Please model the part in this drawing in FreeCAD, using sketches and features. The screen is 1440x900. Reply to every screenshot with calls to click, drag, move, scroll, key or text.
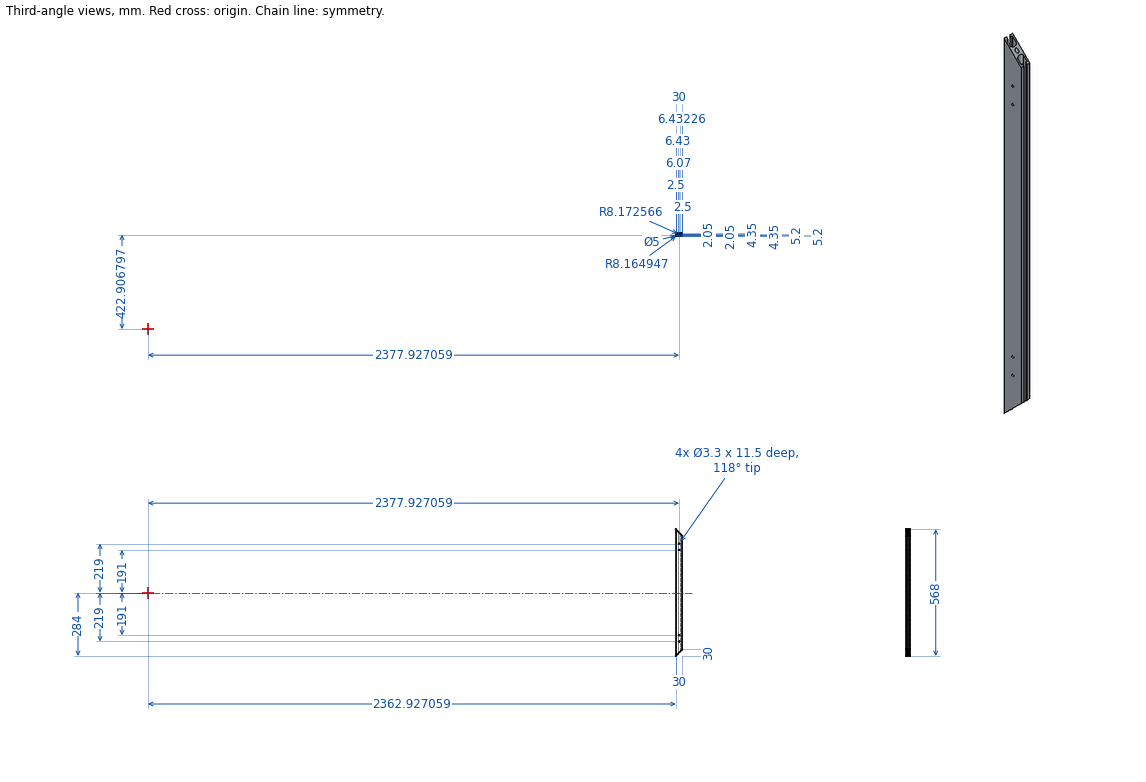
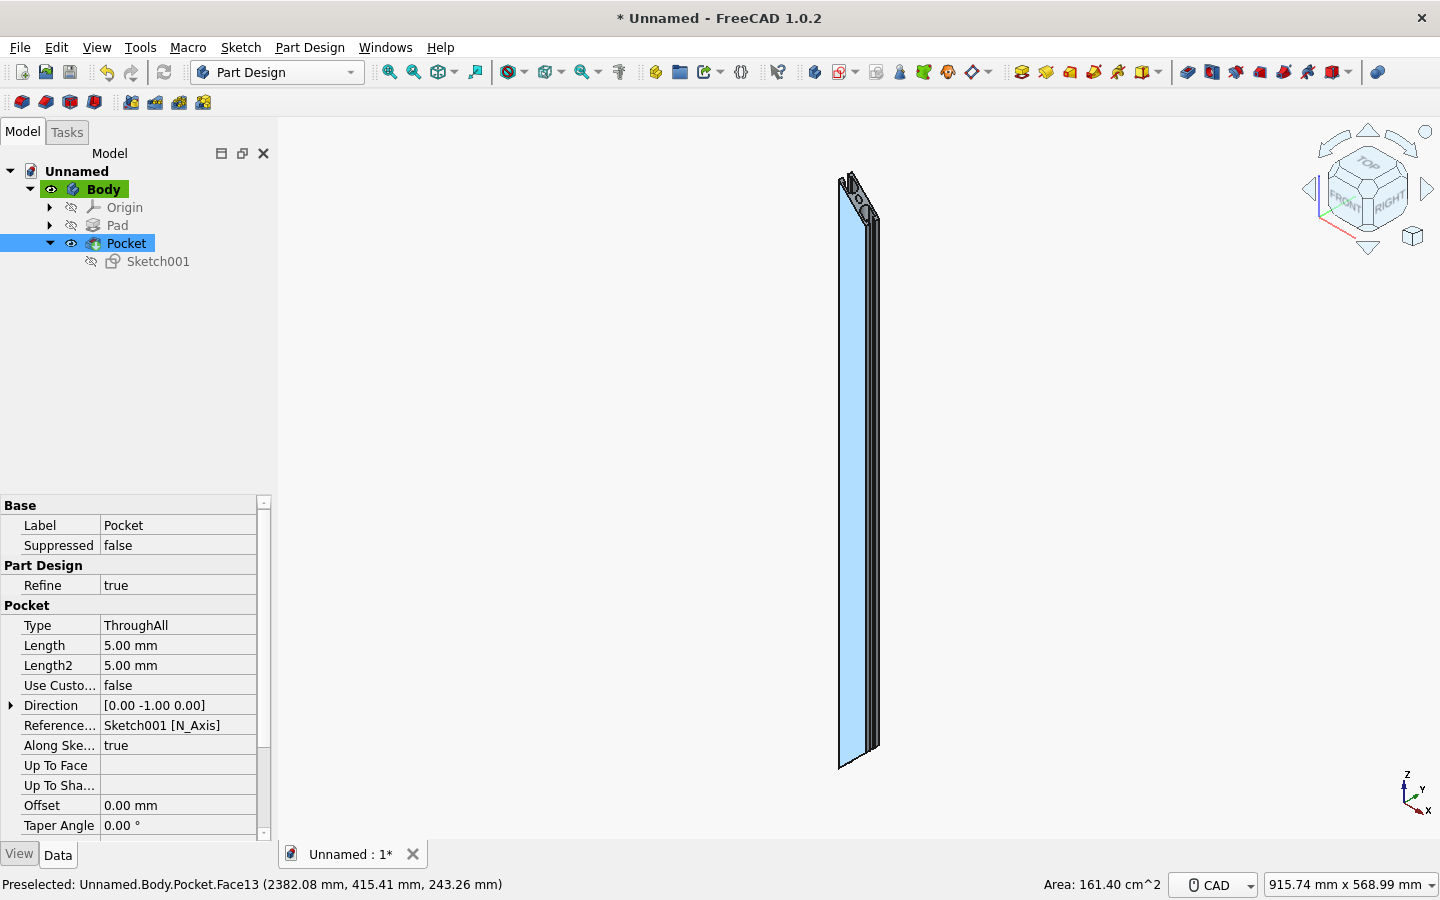
click(840, 72)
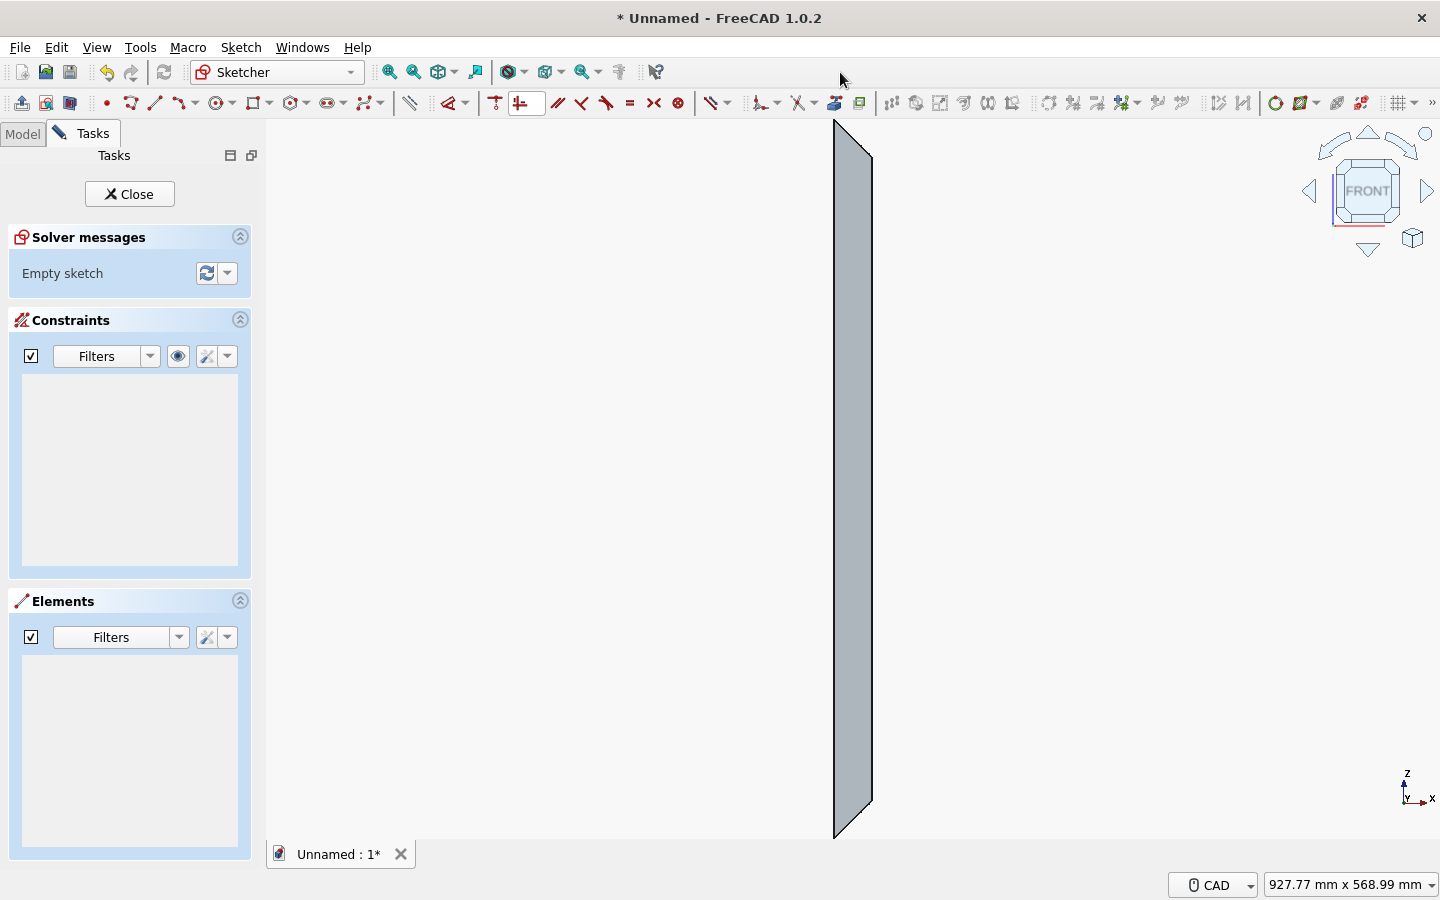
click(216, 104)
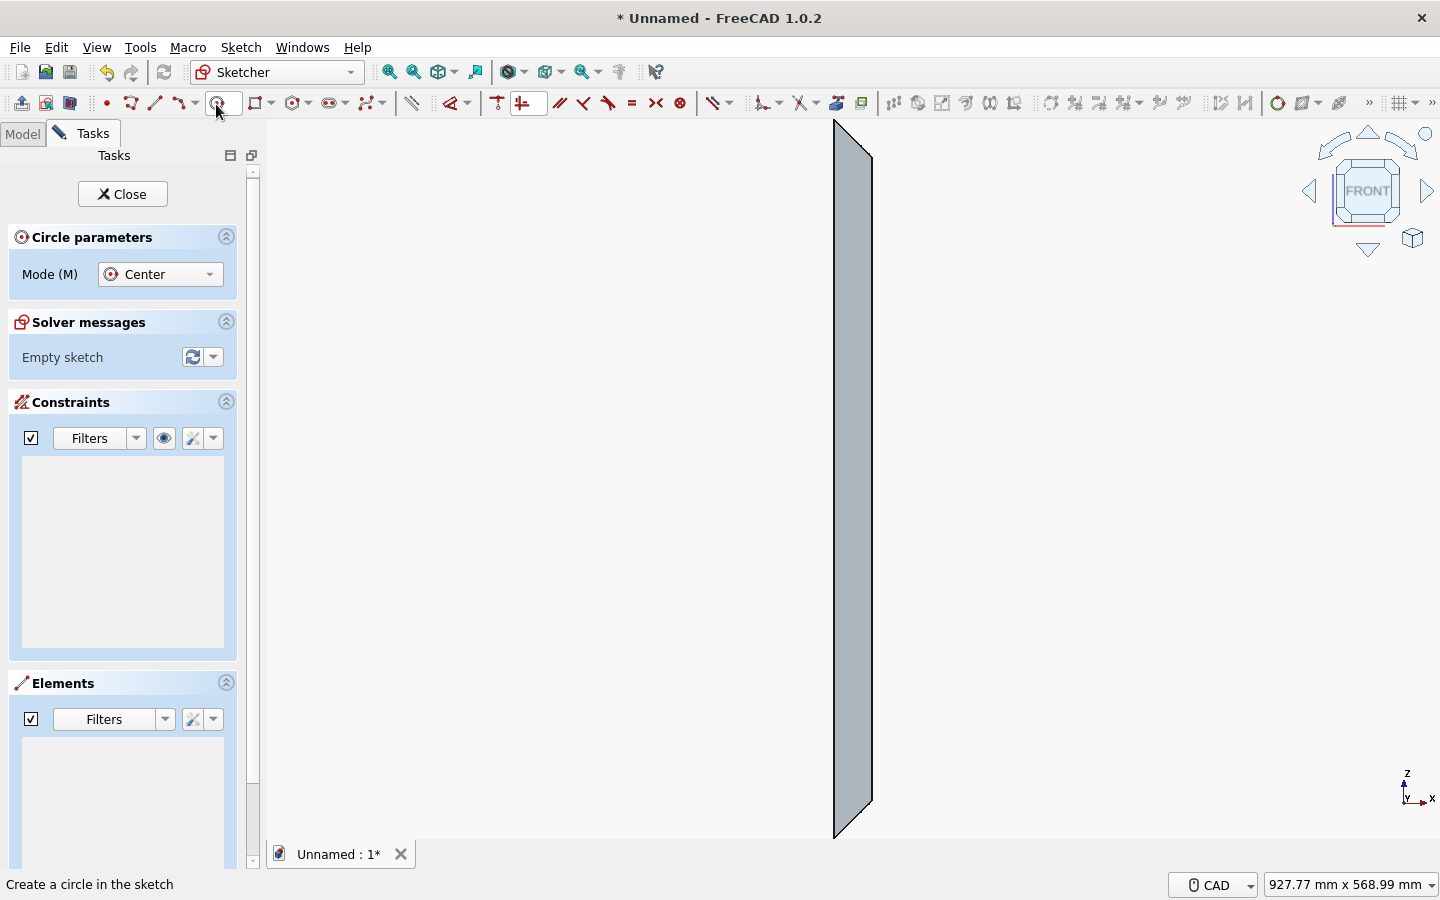
scroll(853, 202, up, 12)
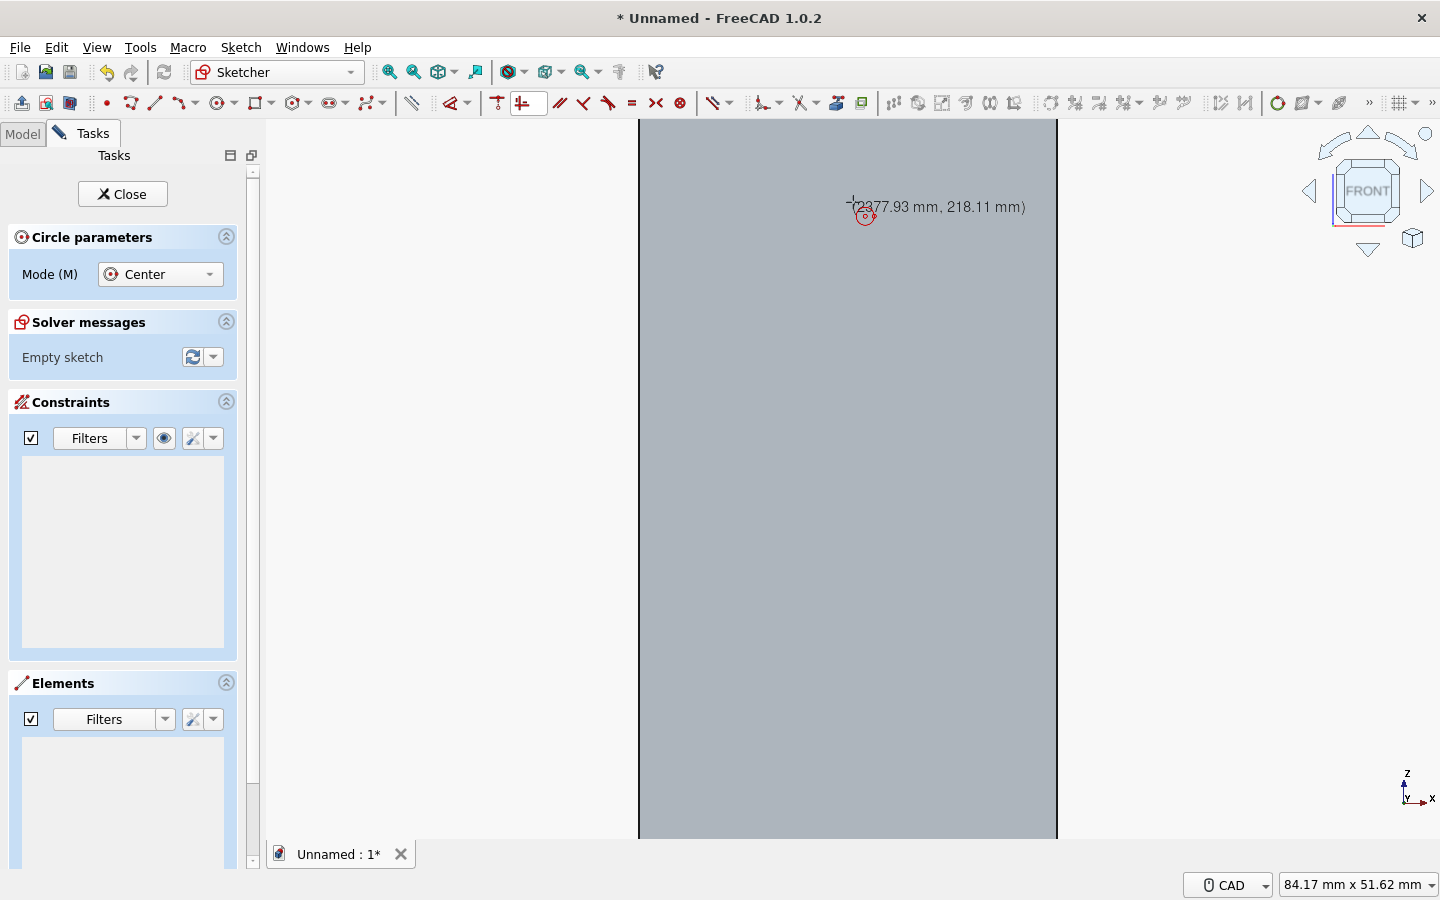
scroll(779, 256, down, 13)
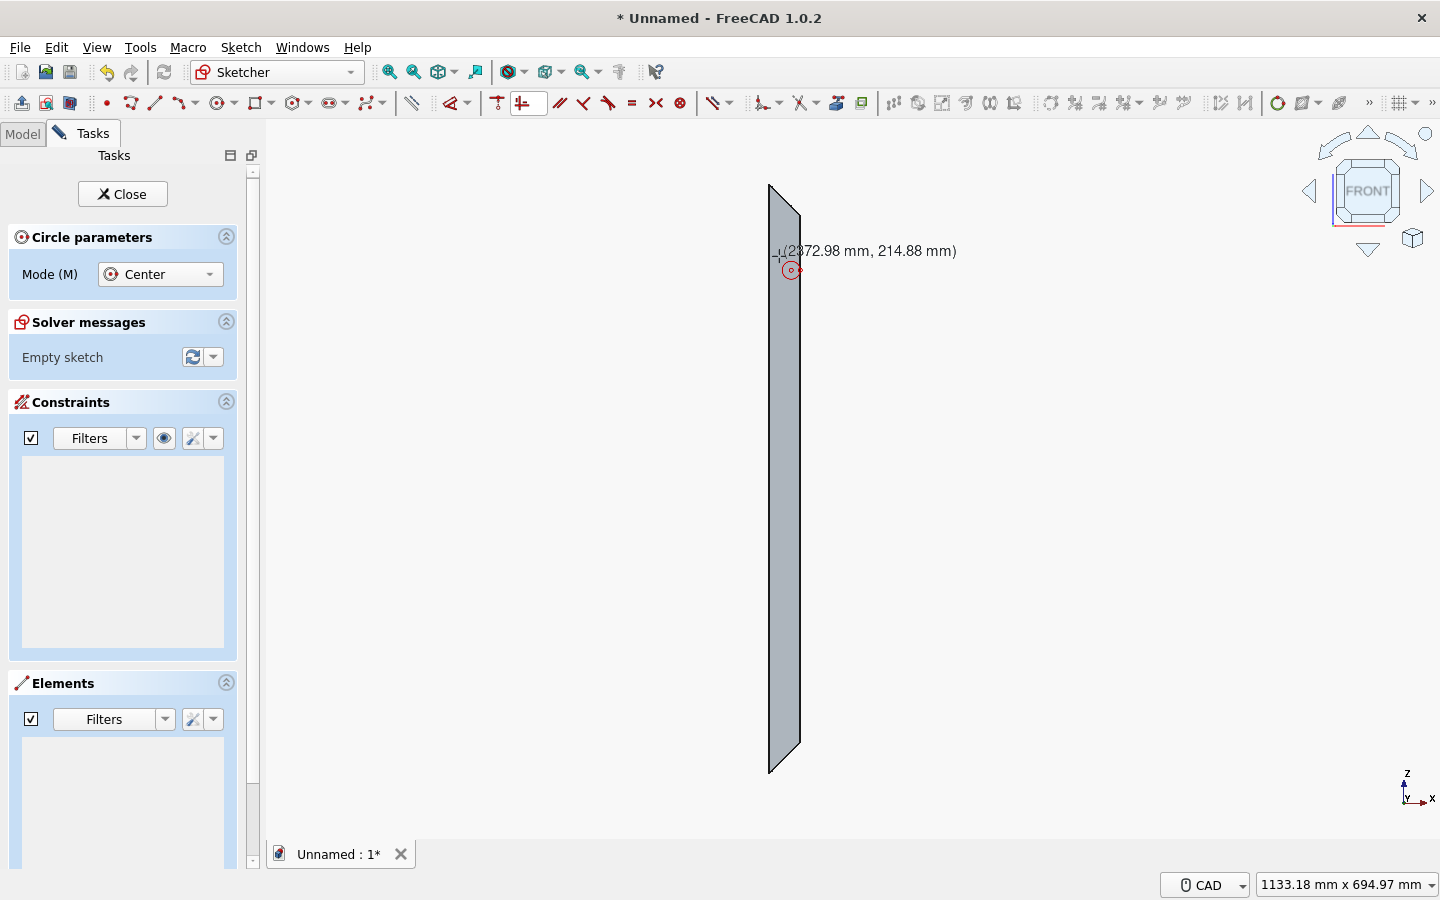
click(785, 252)
move(786, 251)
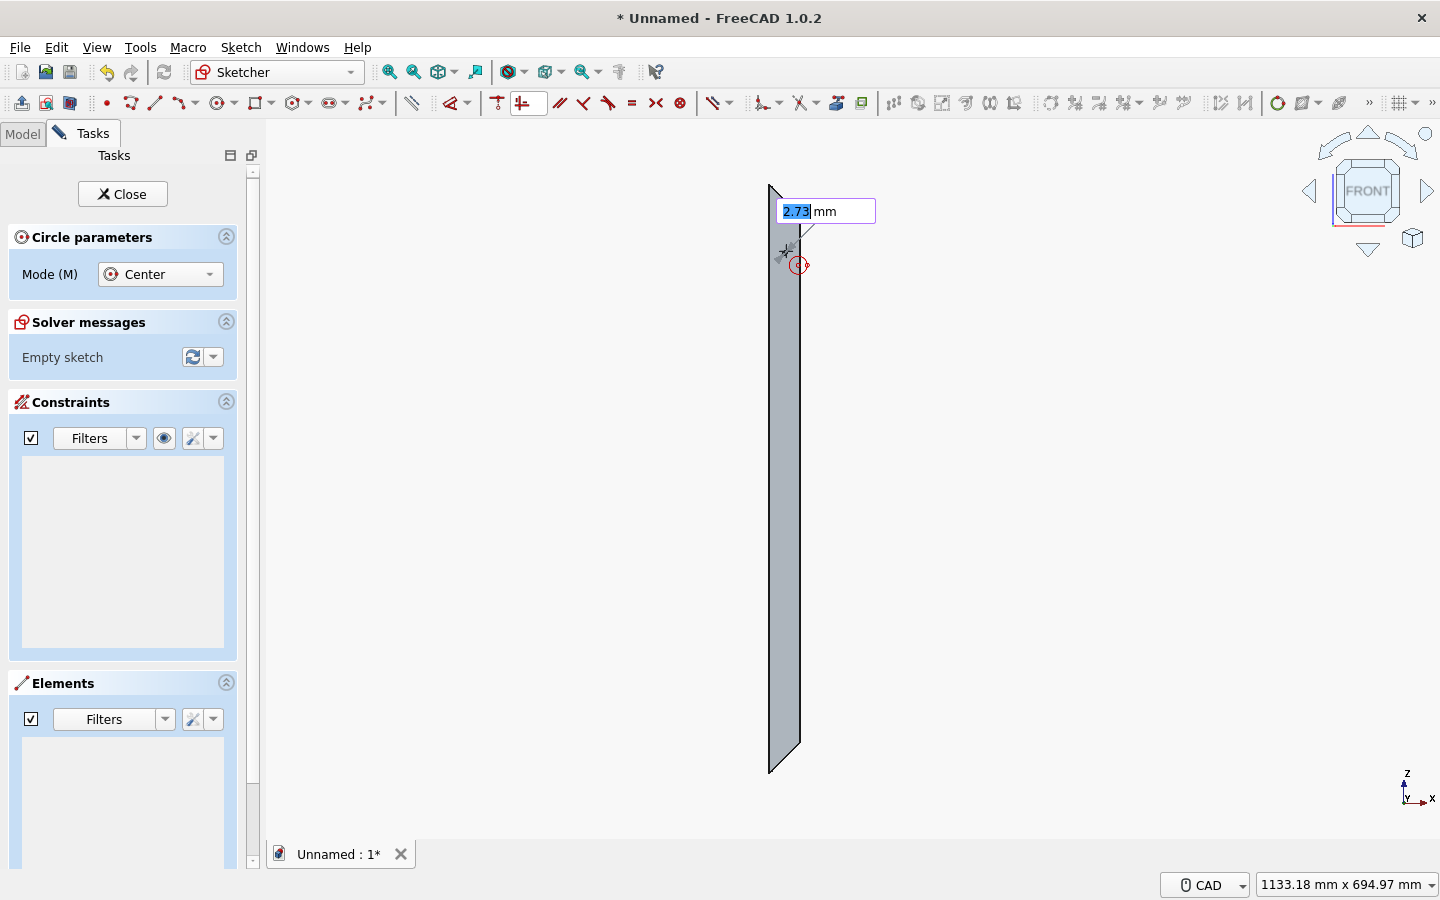
text(3.3)
key(Return)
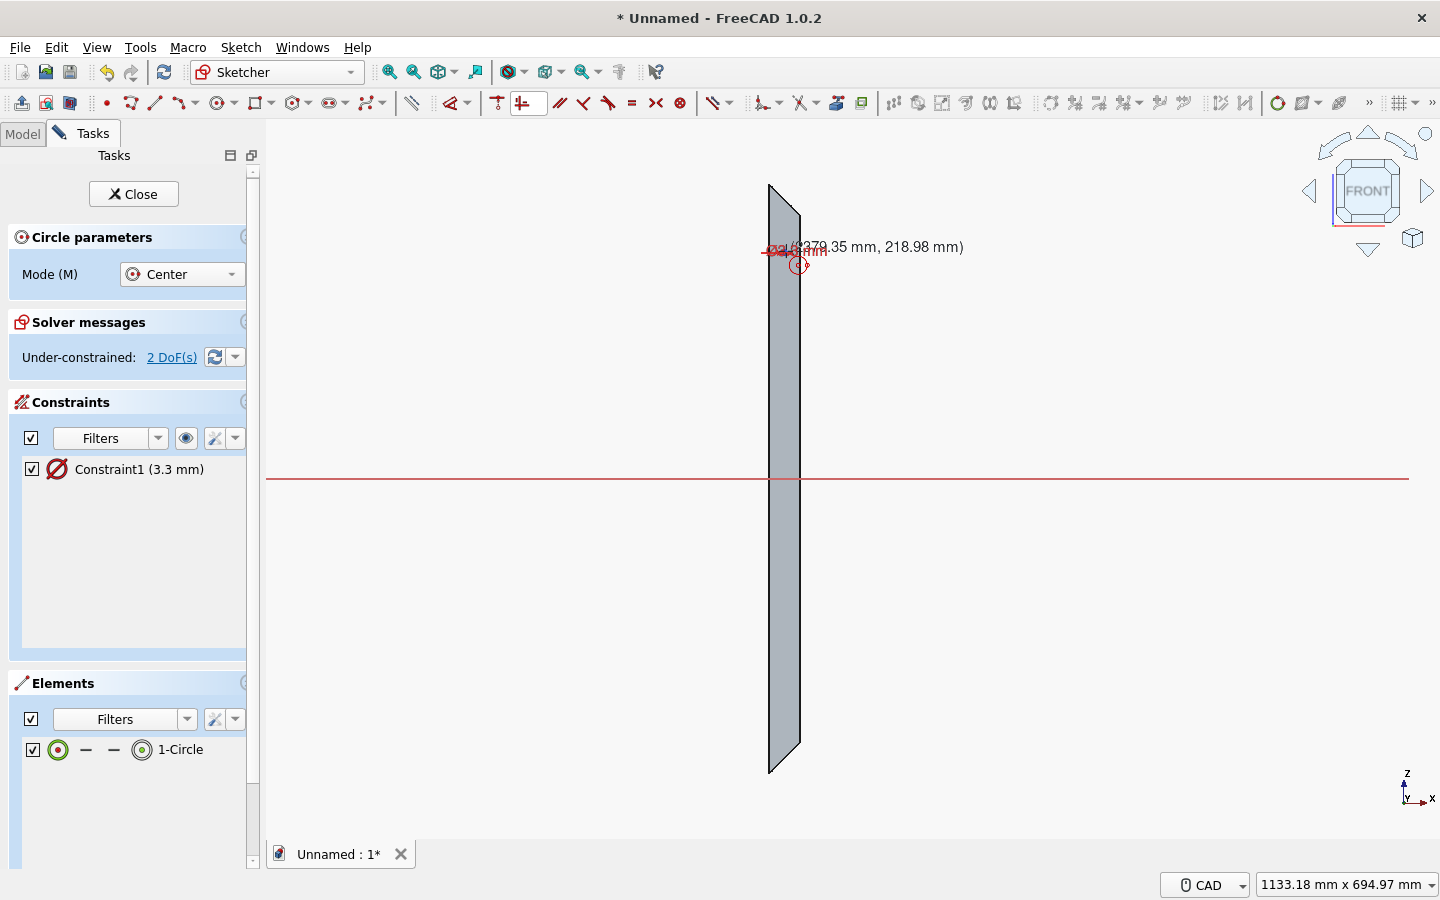
scroll(785, 281, up, 13)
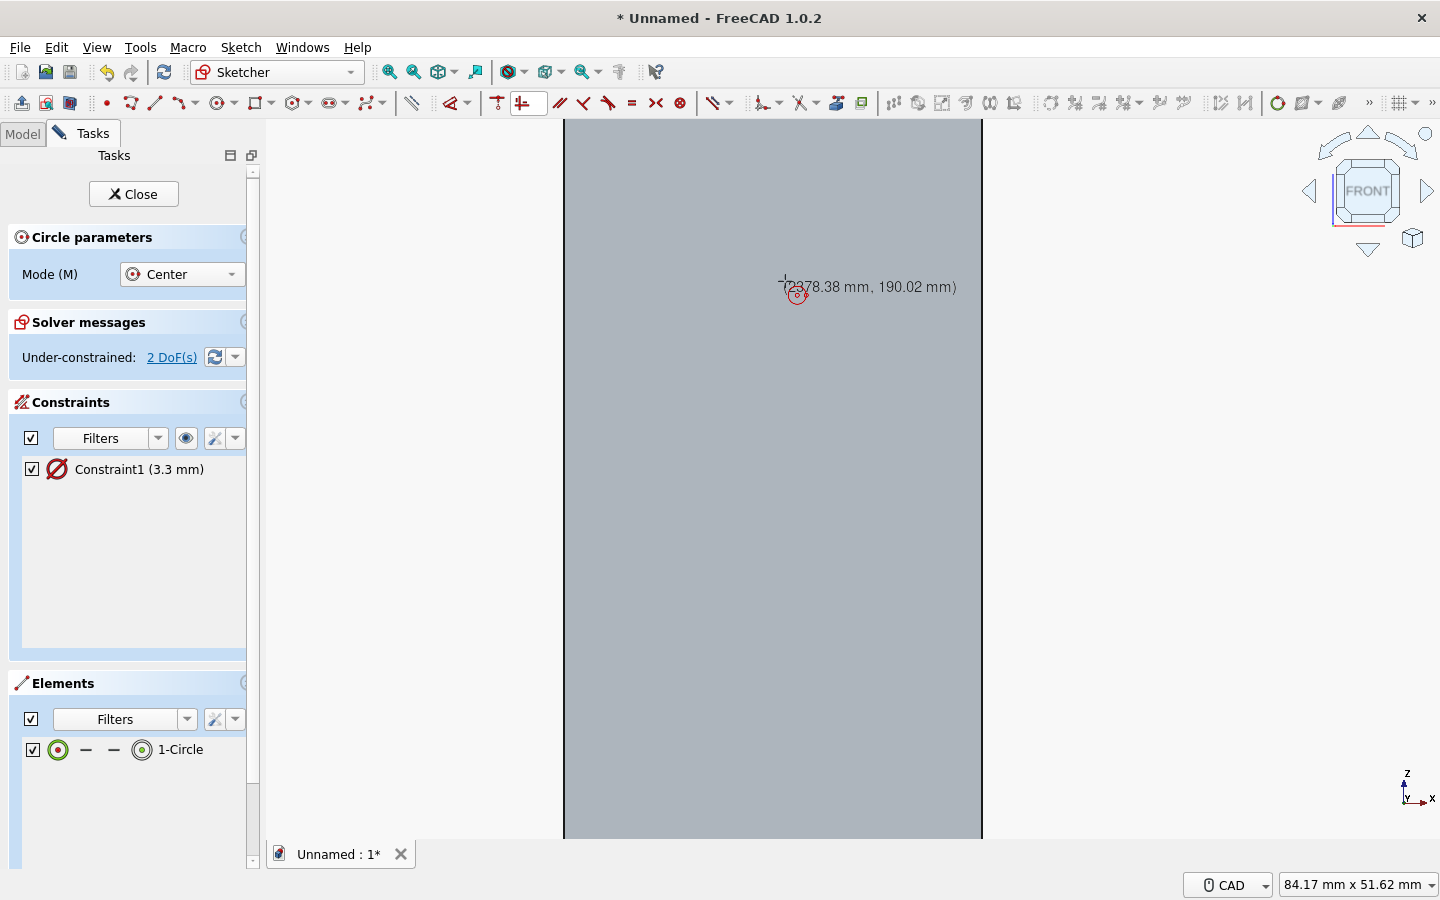
scroll(785, 281, down, 13)